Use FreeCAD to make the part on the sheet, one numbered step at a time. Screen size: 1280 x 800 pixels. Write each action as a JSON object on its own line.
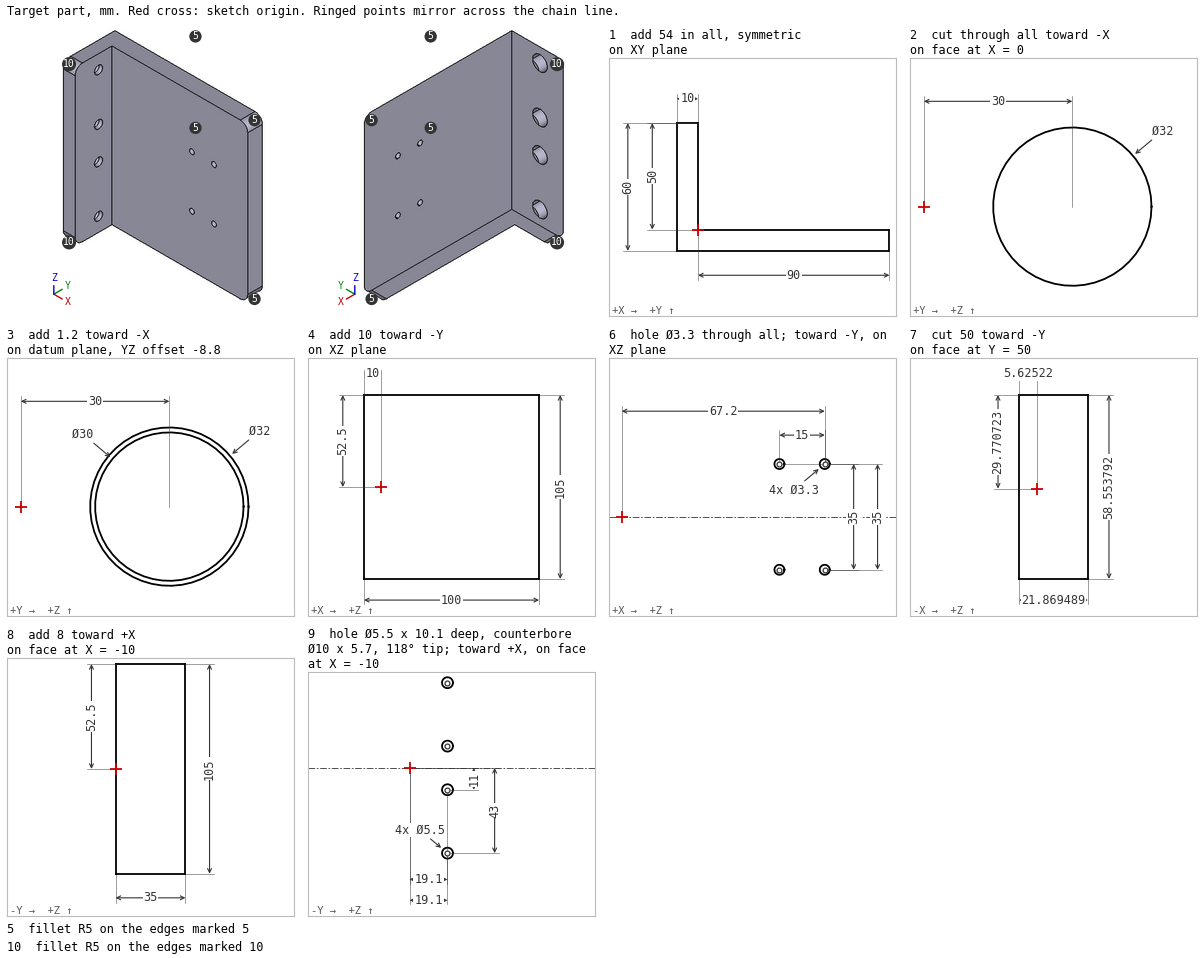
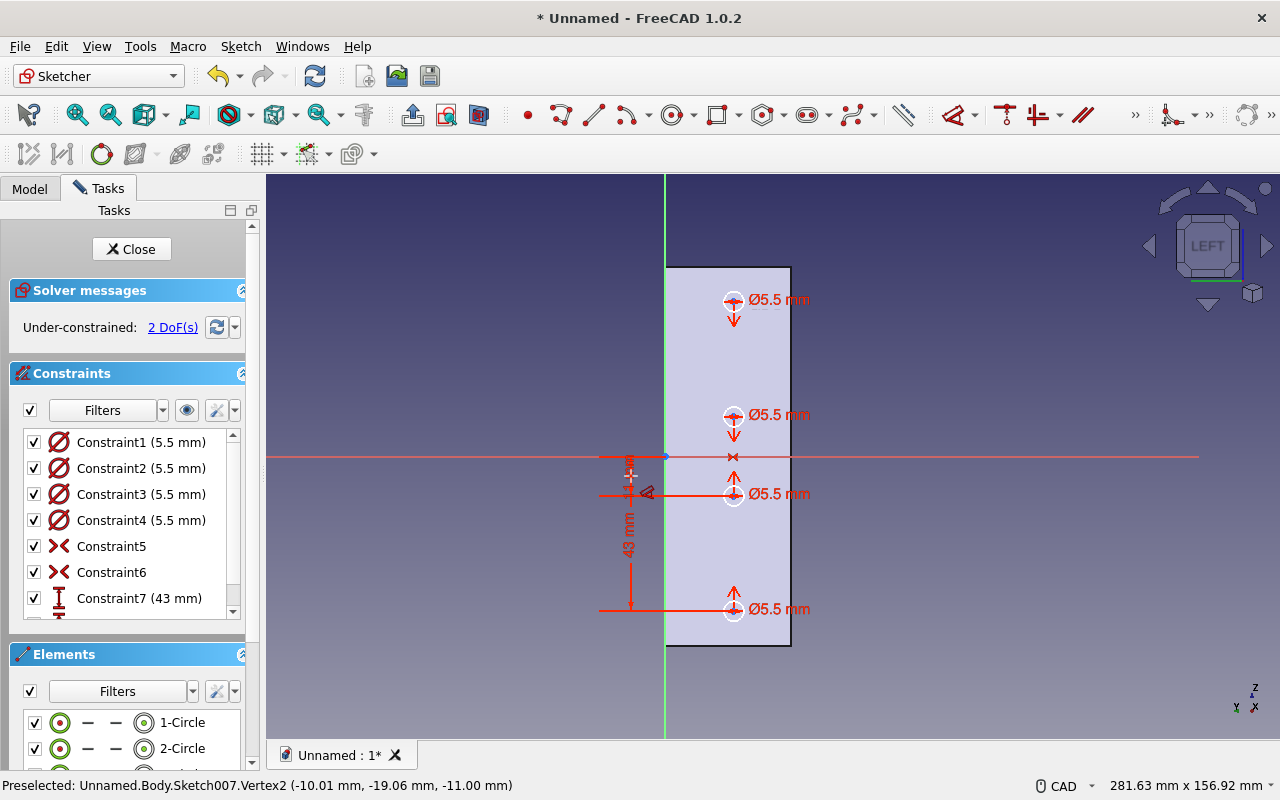
{"action": "left_click", "coordinate": [734, 611]}
{"action": "left_click", "coordinate": [700, 645]}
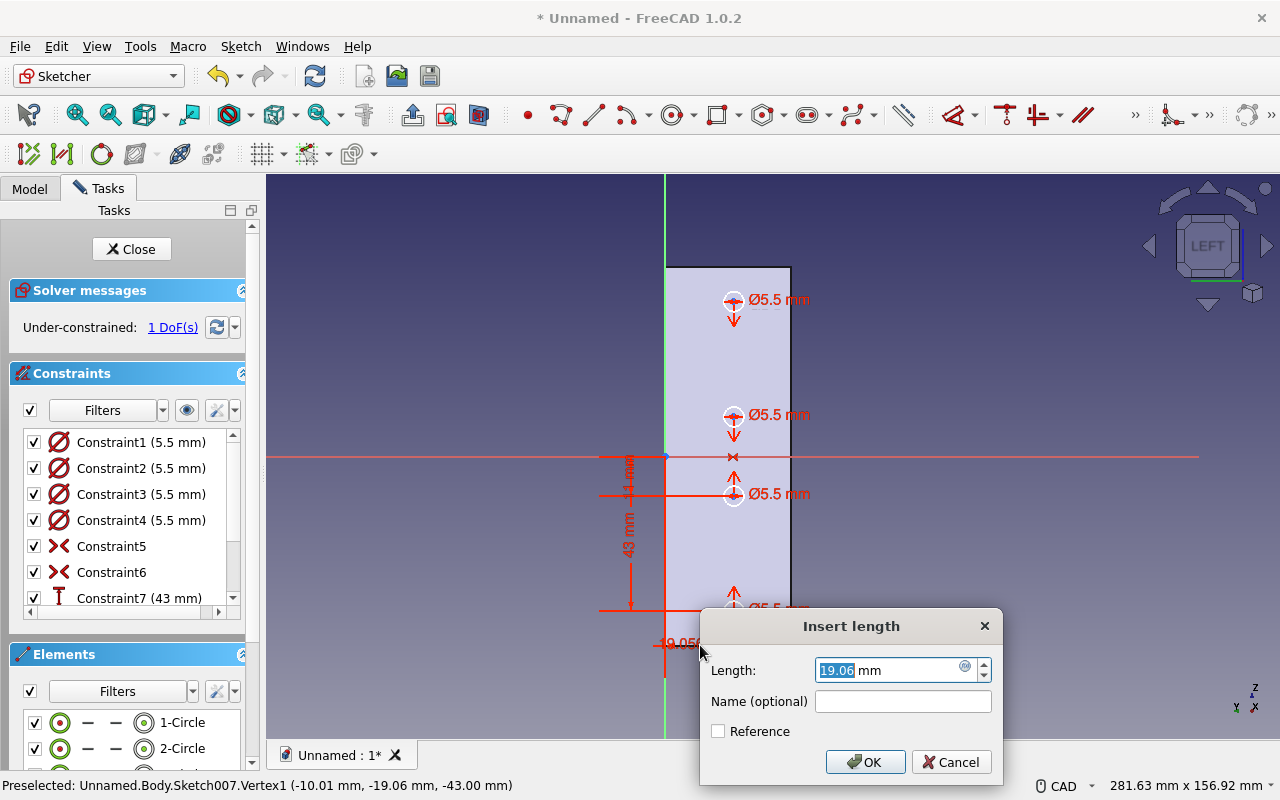
{"action": "type", "text": "19.1"}
{"action": "key", "text": "Return"}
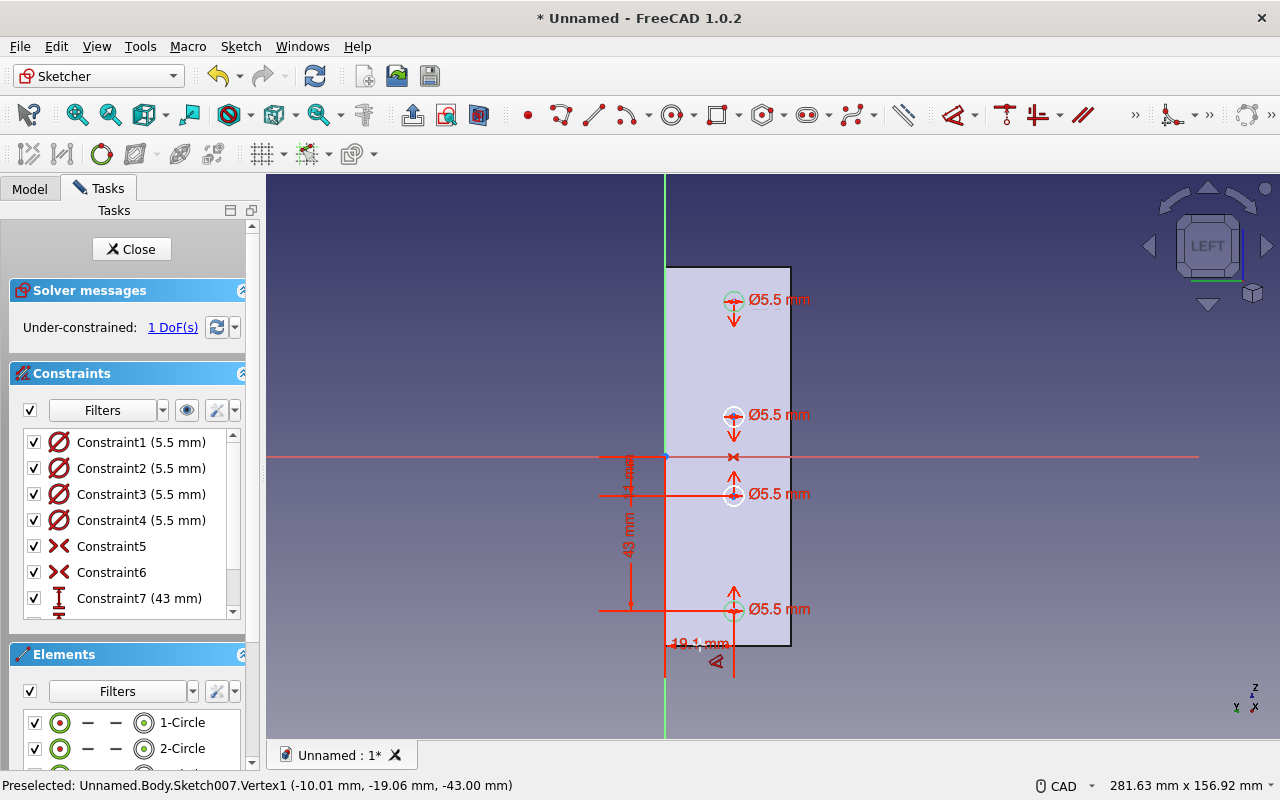
{"action": "left_click", "coordinate": [734, 496]}
{"action": "left_click", "coordinate": [715, 530]}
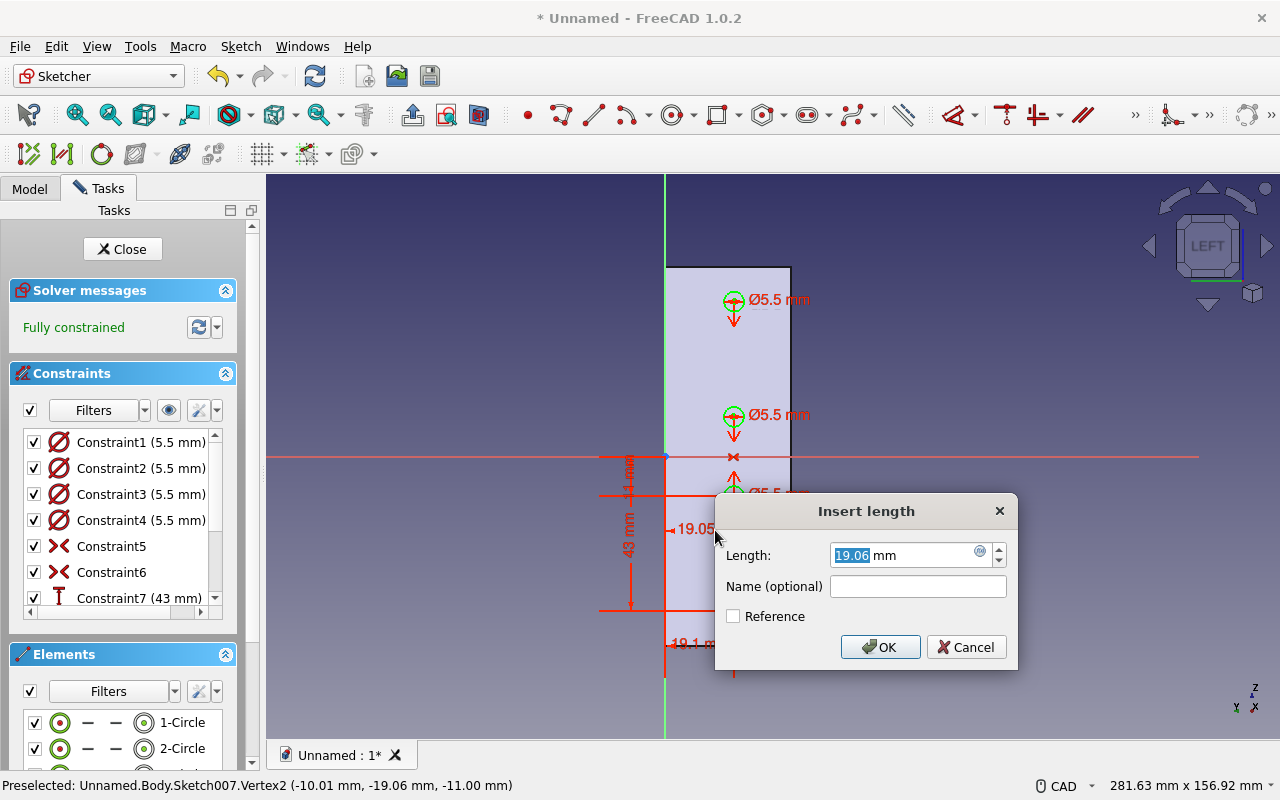
{"action": "type", "text": "19.1"}
{"action": "key", "text": "Return"}
{"action": "key", "text": "Escape"}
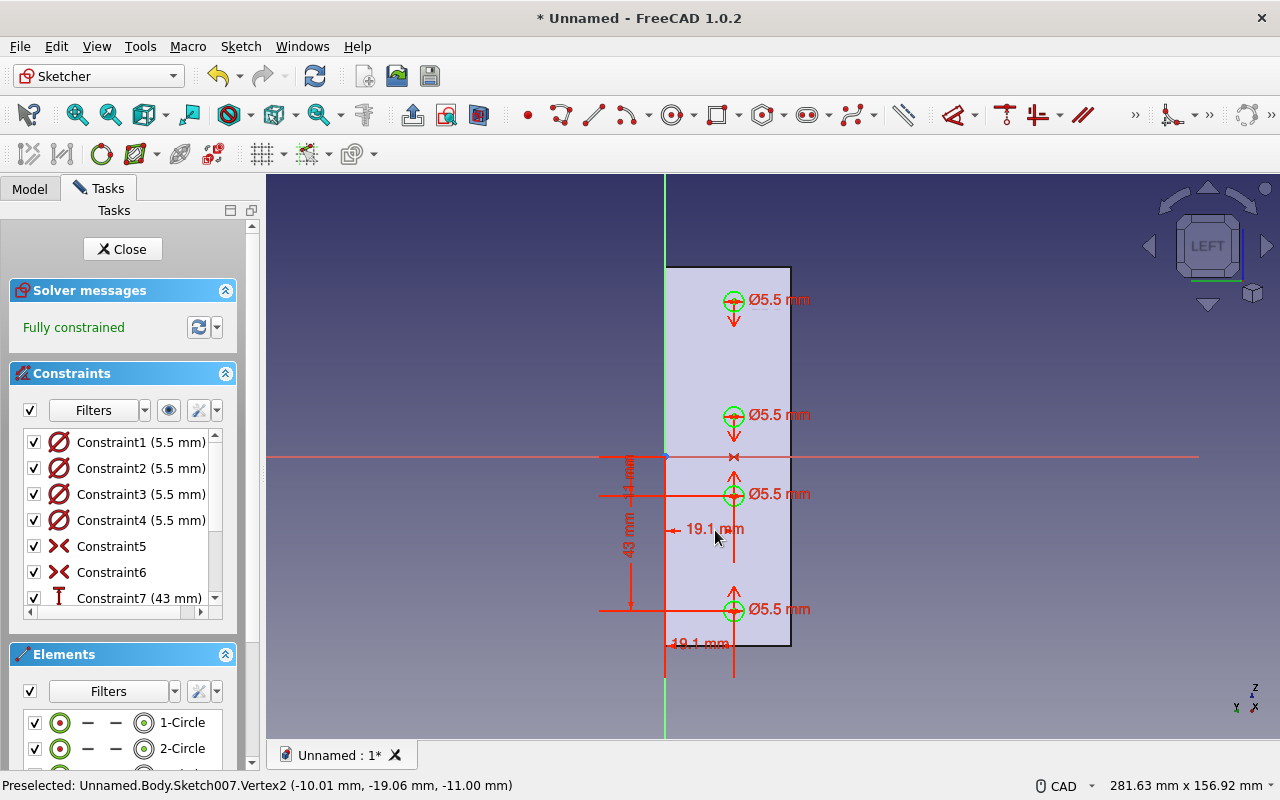
{"action": "left_click", "coordinate": [123, 249]}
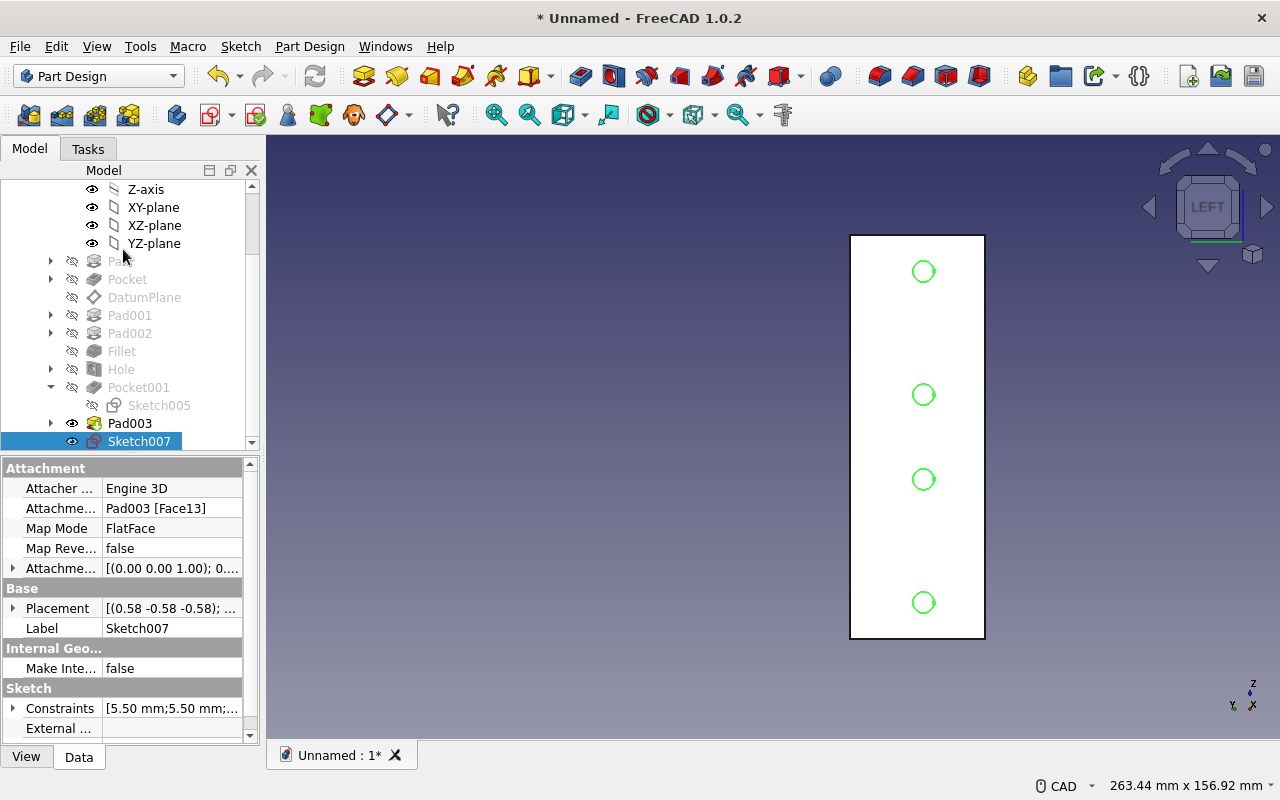
{"action": "left_click", "coordinate": [614, 76]}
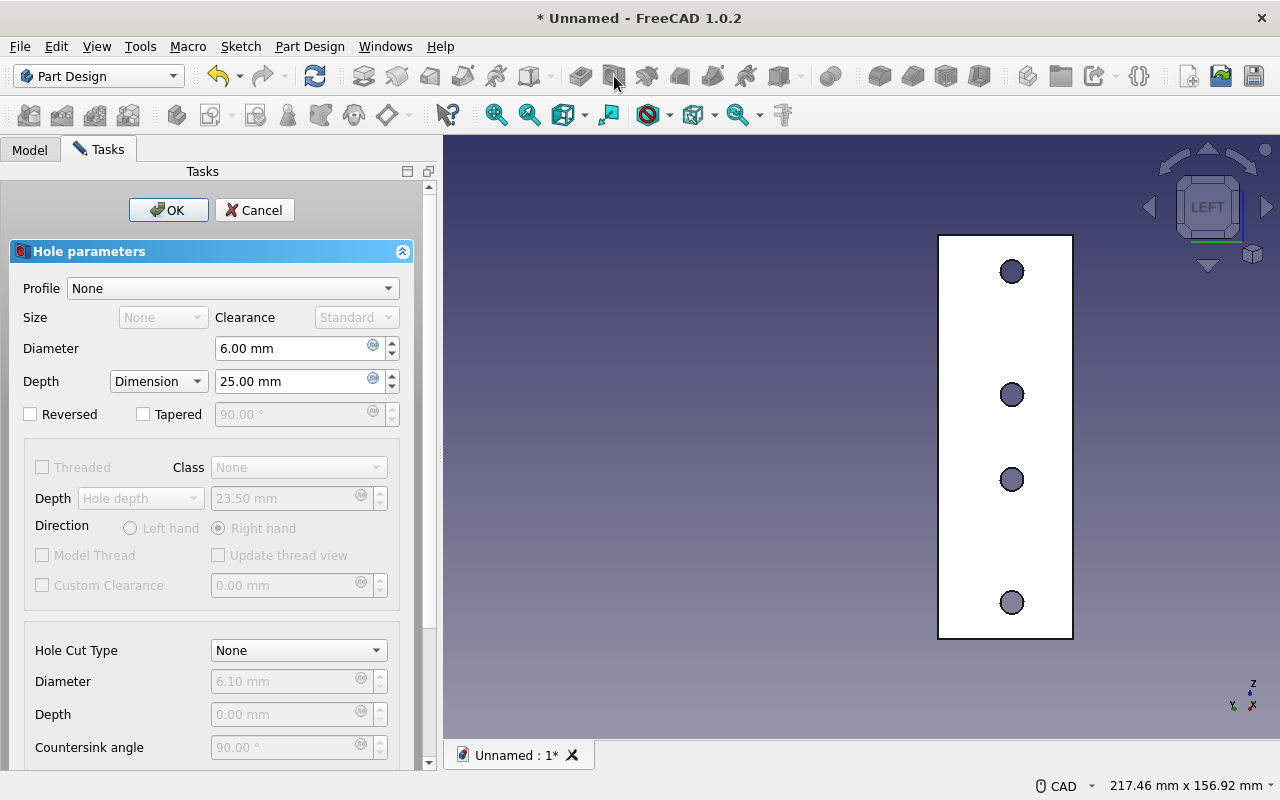
{"action": "triple_click", "coordinate": [300, 348]}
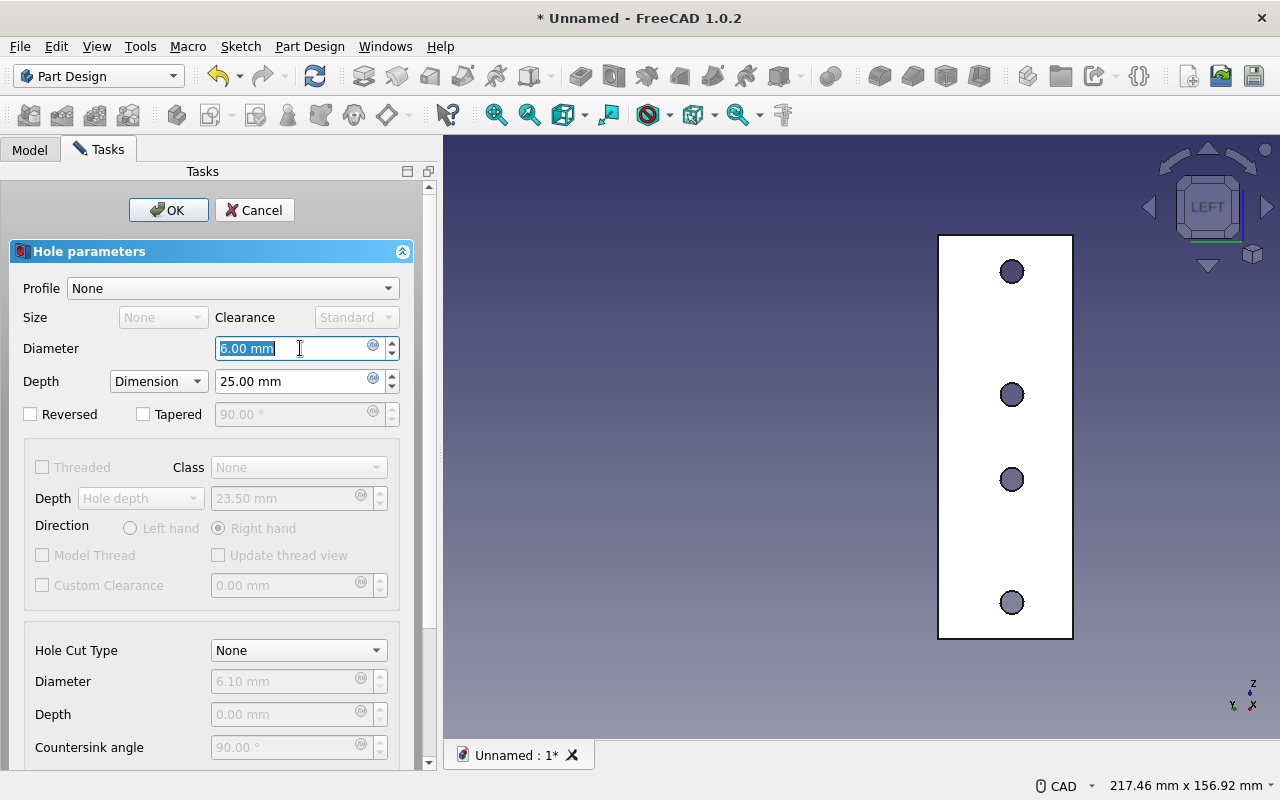
{"action": "type", "text": "5.5"}
{"action": "key", "text": "Tab"}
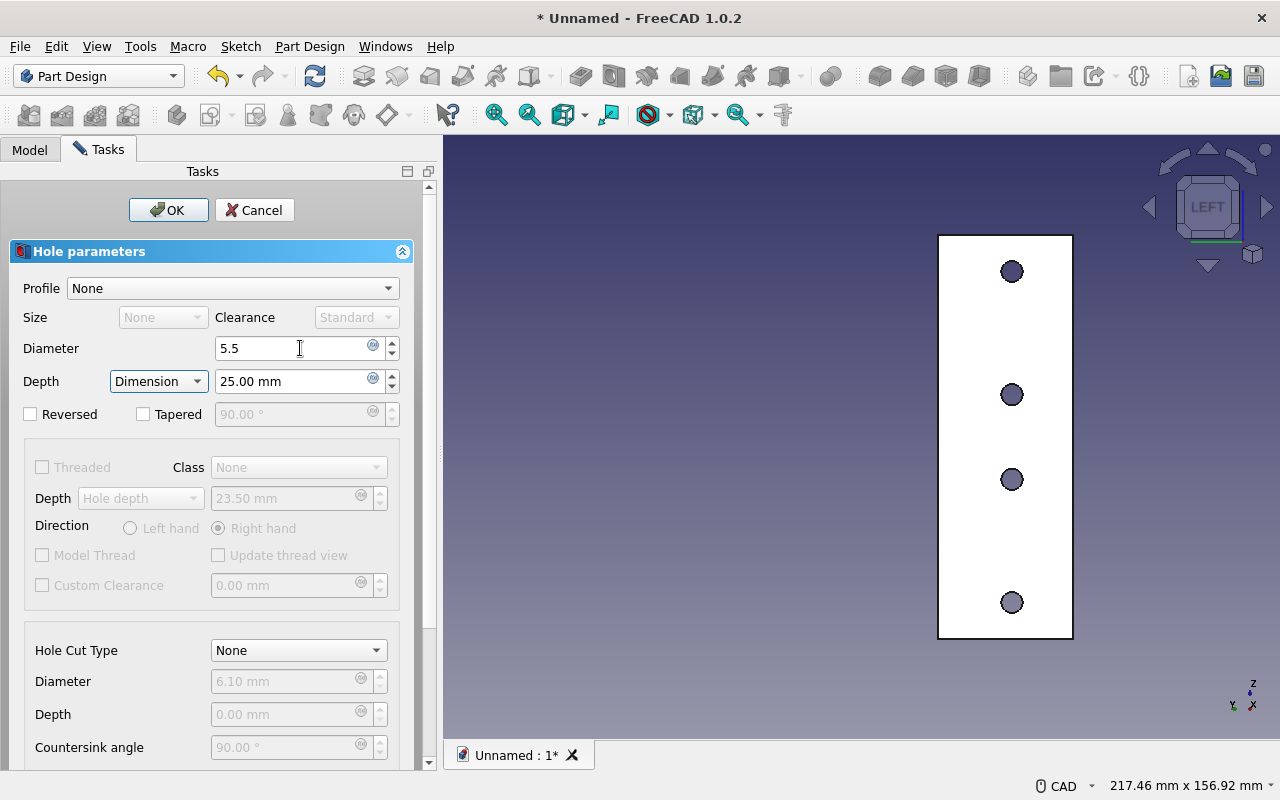
{"action": "triple_click", "coordinate": [300, 382]}